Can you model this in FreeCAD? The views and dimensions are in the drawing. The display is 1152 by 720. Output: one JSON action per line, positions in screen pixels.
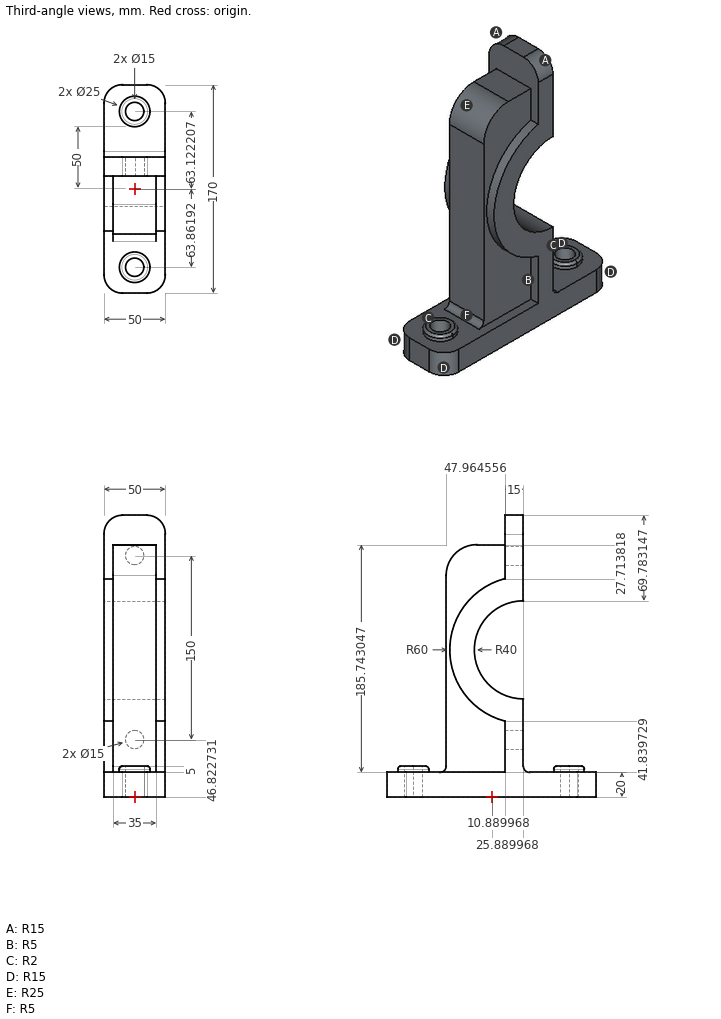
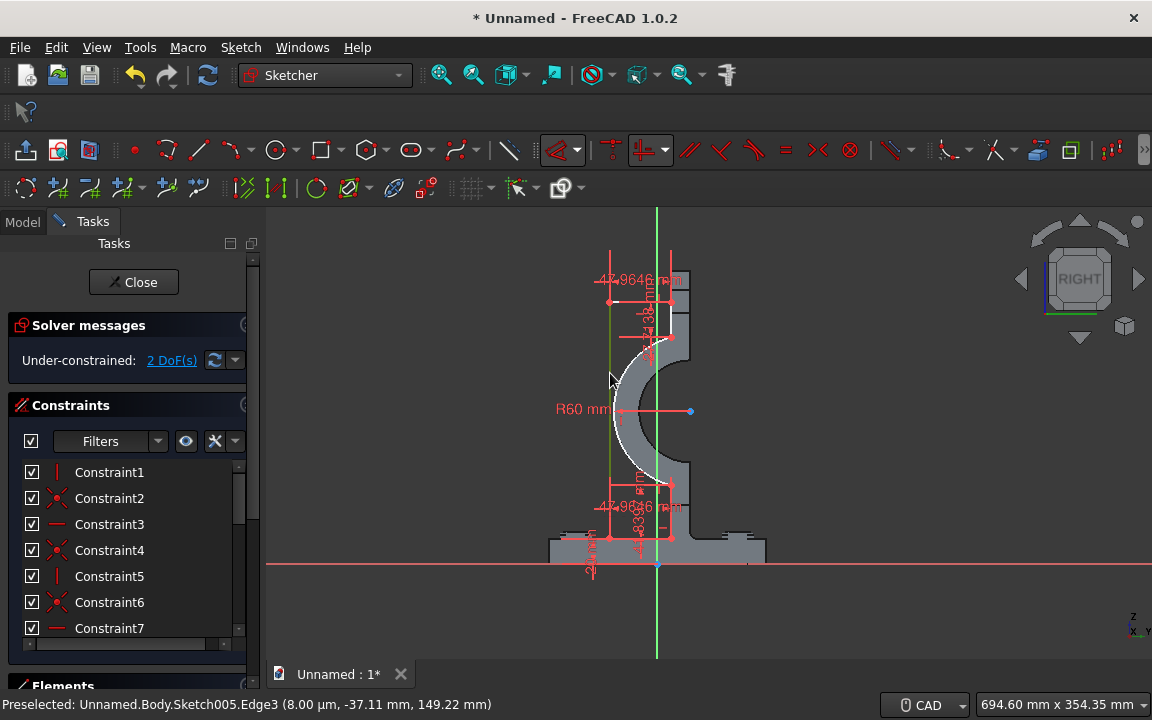
{"action": "key", "text": "i"}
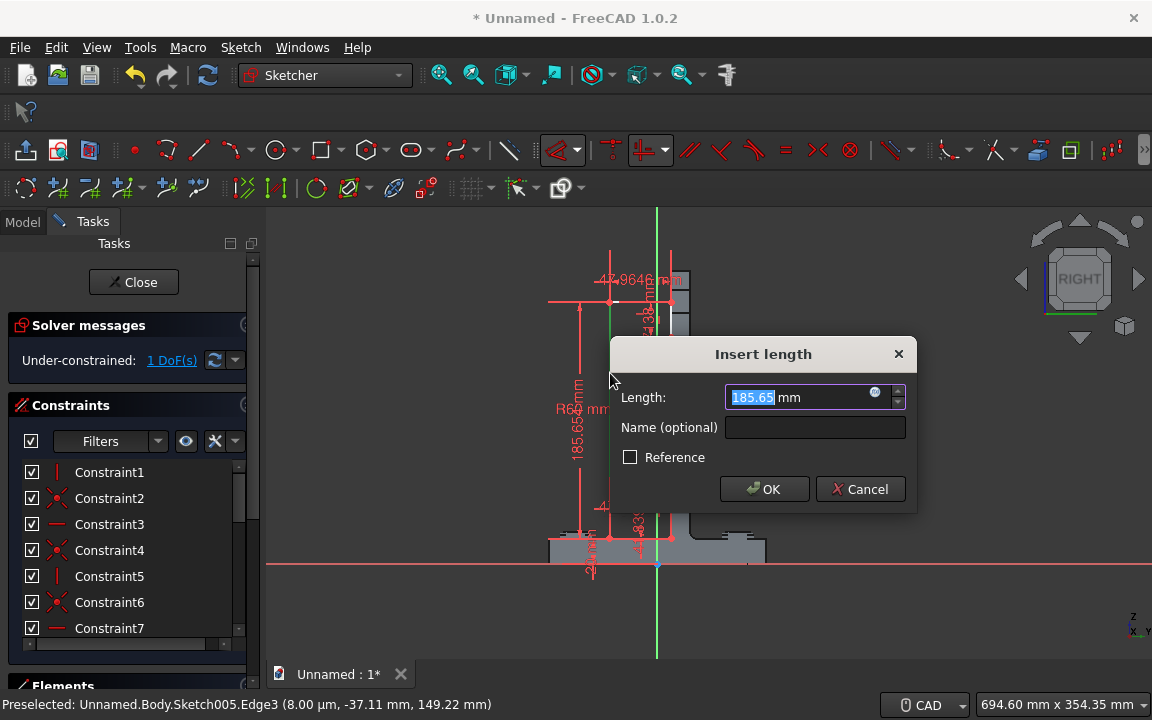
{"action": "type", "text": "185.743047"}
{"action": "key", "text": "Return"}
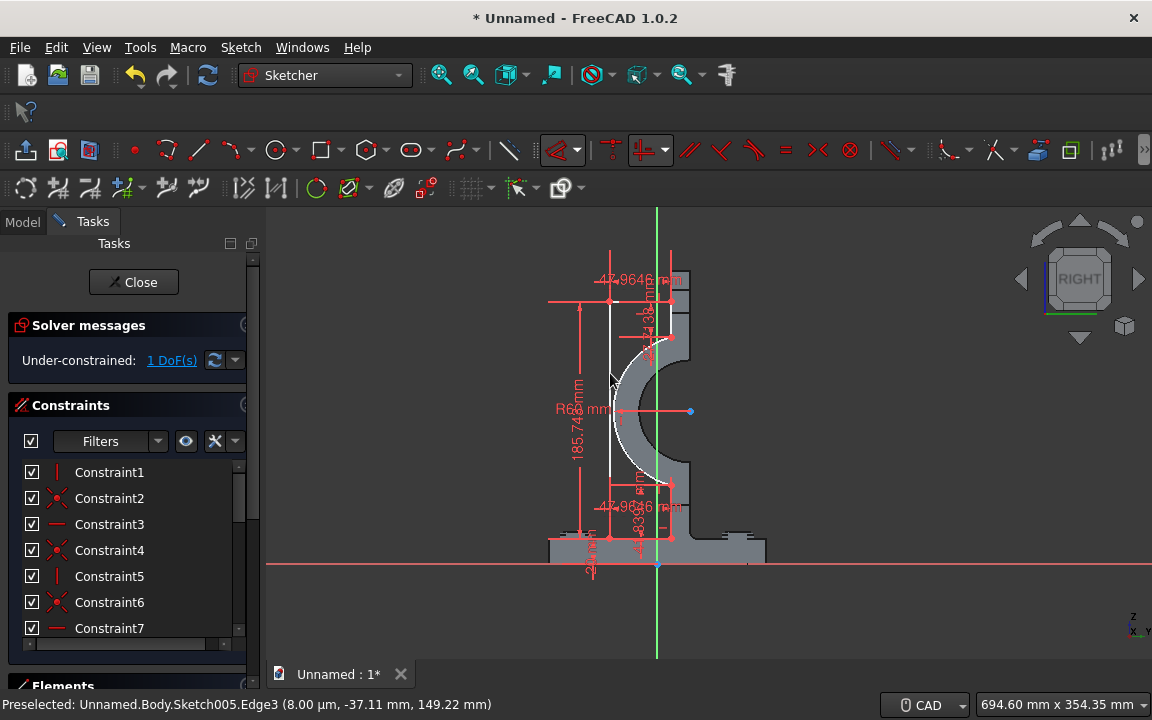
{"action": "scroll", "coordinate": [671, 337], "scroll_direction": "up", "scroll_amount": 6}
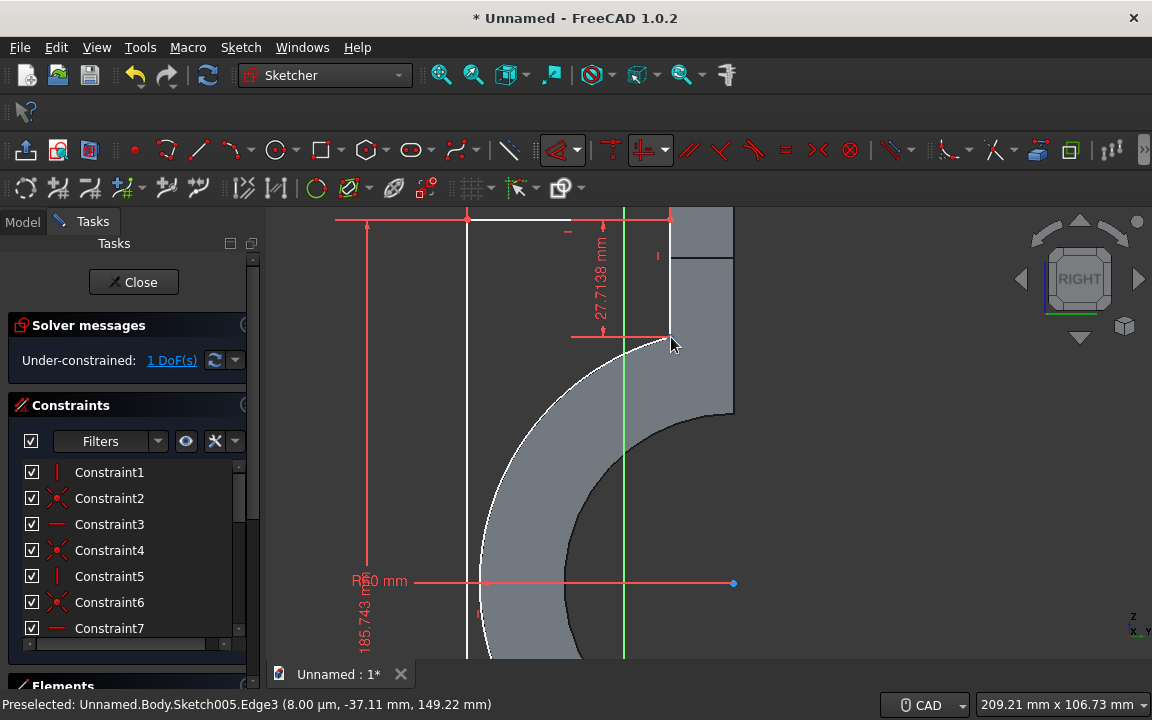
{"action": "left_click", "coordinate": [670, 337]}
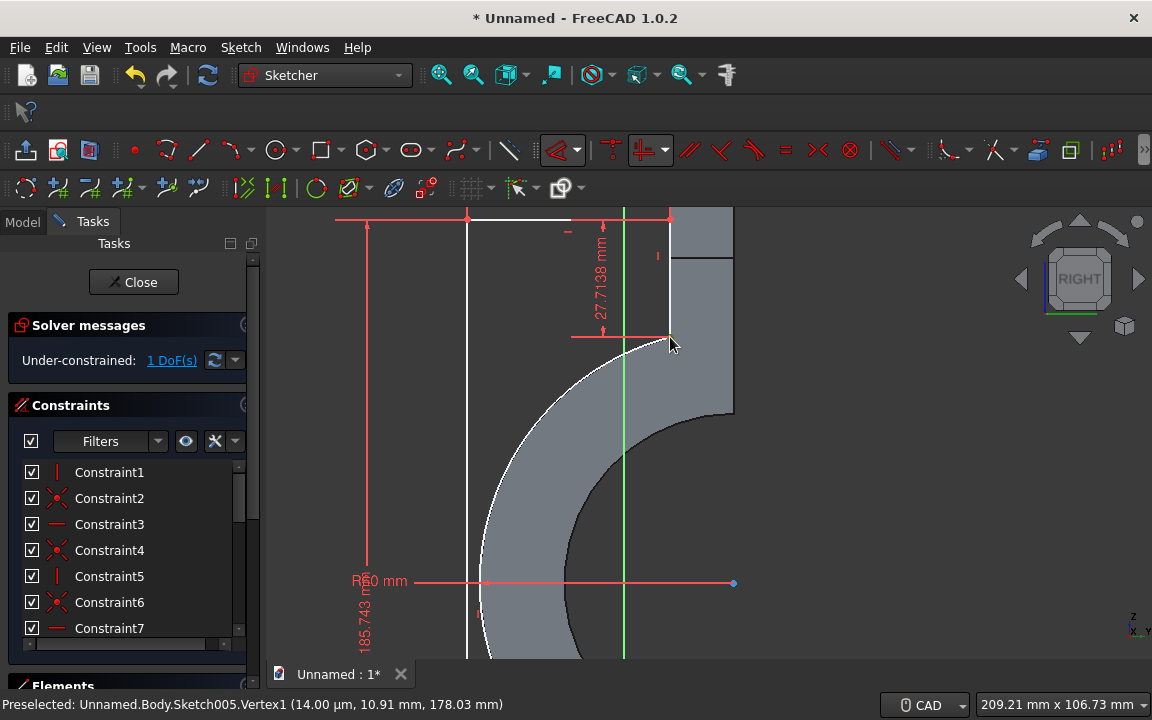
{"action": "key", "text": "l"}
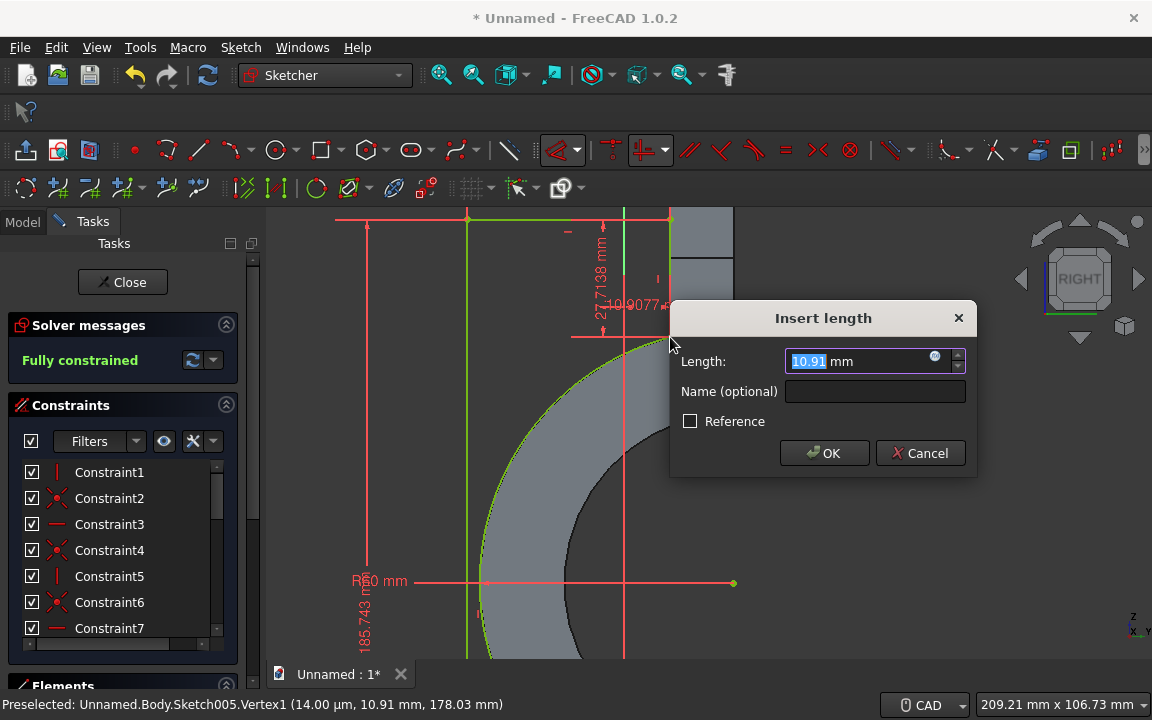
{"action": "type", "text": "10.889968"}
{"action": "key", "text": "Return"}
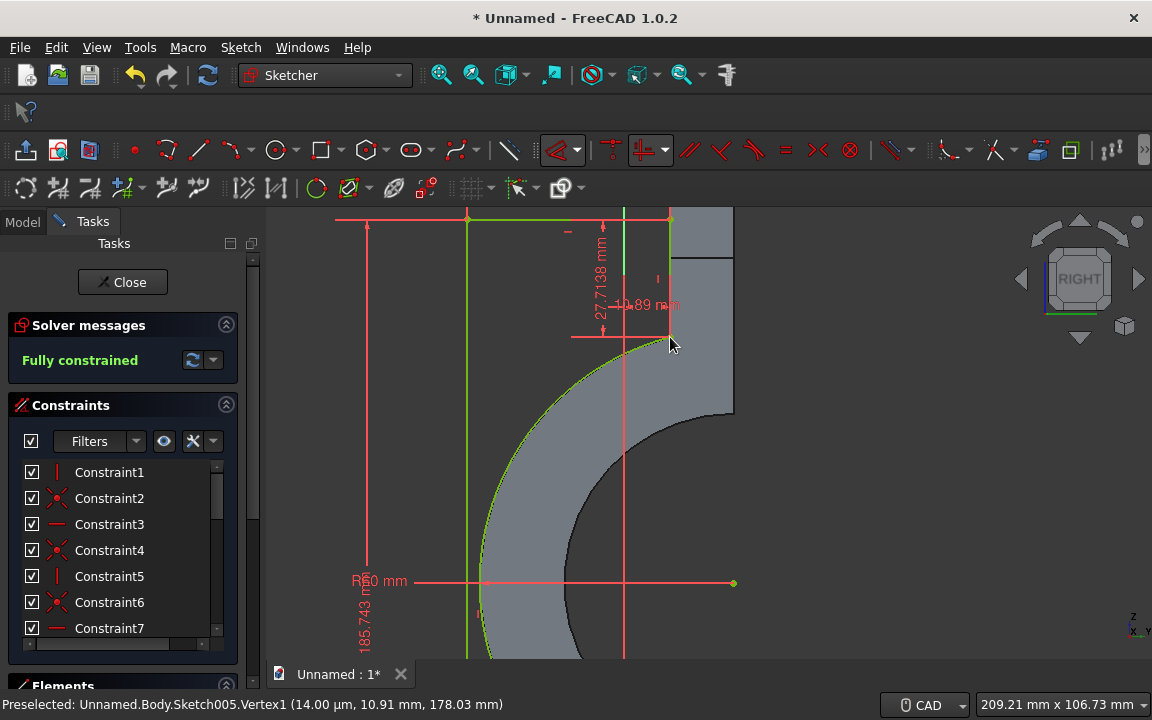
{"action": "left_click", "coordinate": [123, 282]}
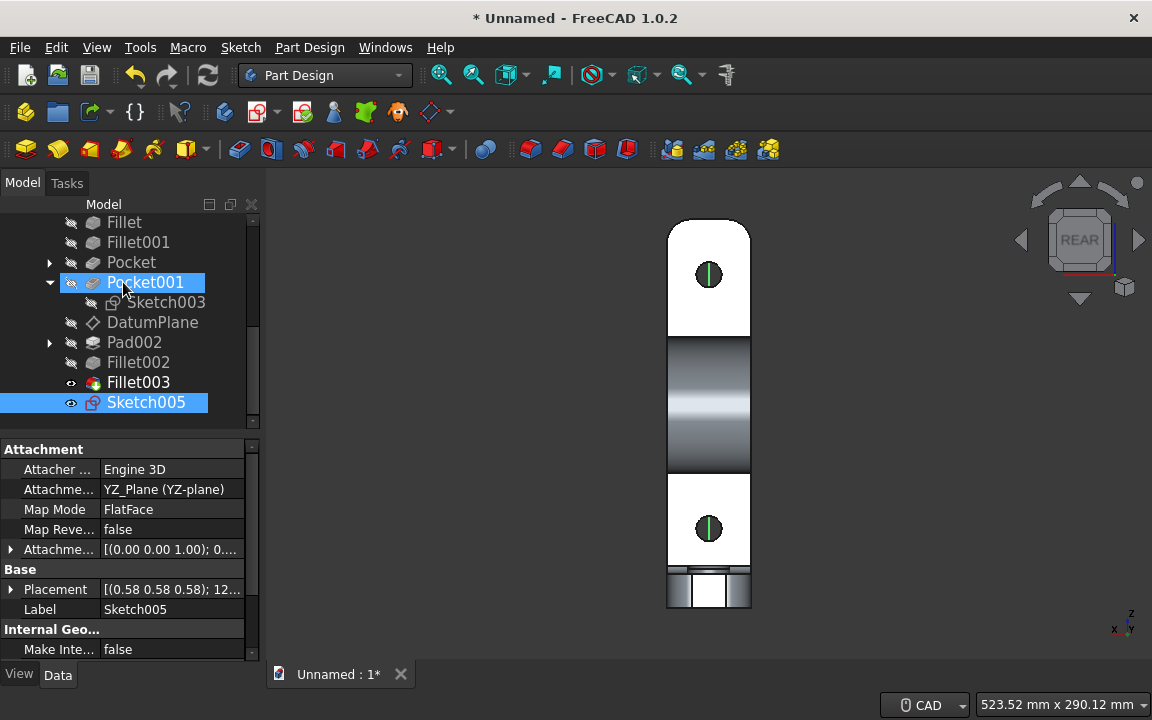
{"action": "left_click", "coordinate": [26, 150]}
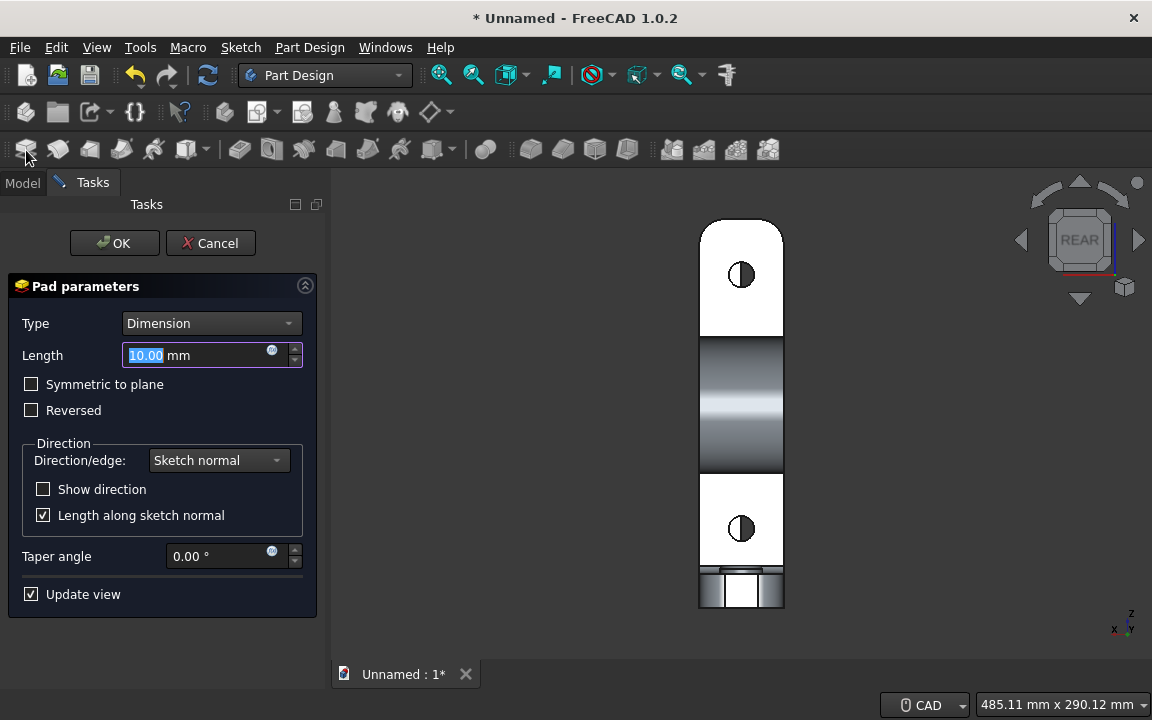
{"action": "type", "text": "35"}
{"action": "key", "text": "Tab"}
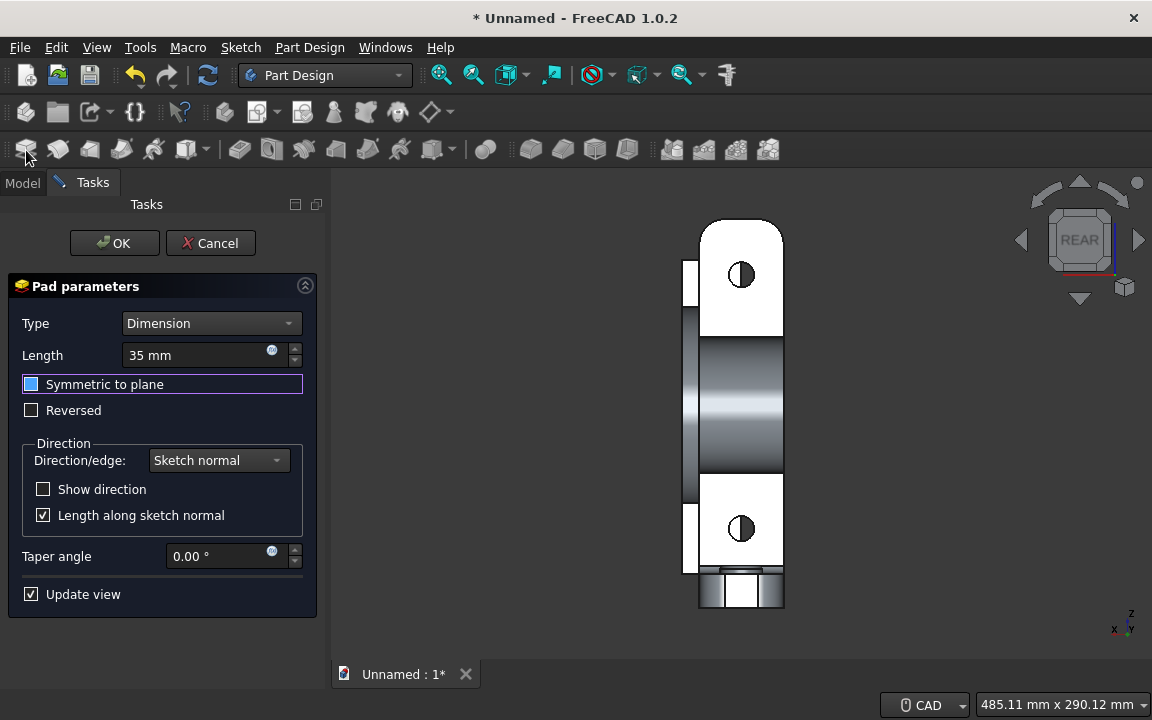
{"action": "left_click", "coordinate": [30, 384]}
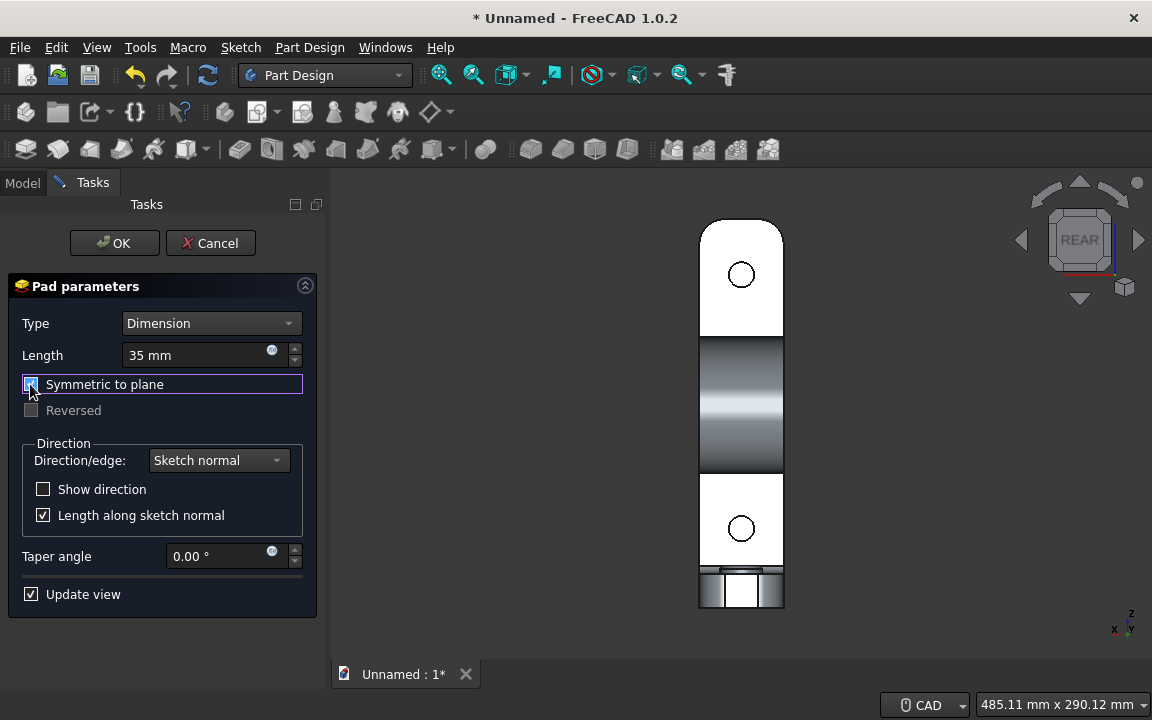
{"action": "left_click", "coordinate": [115, 243]}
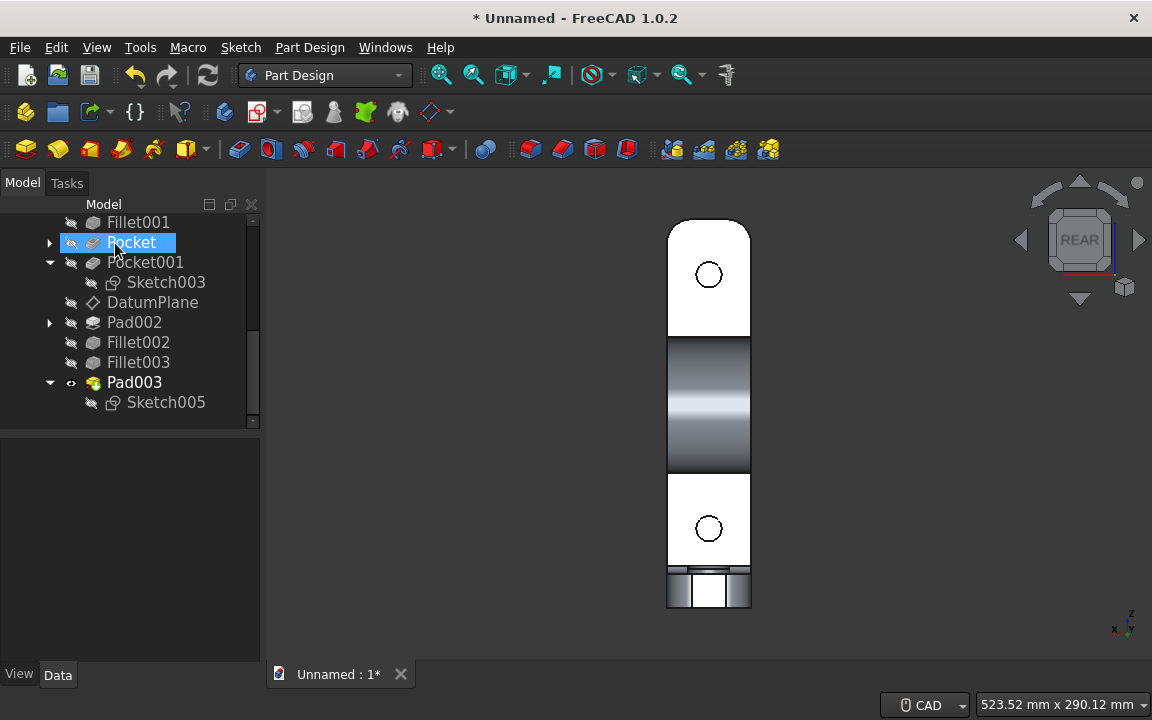
{"action": "key", "text": "0"}